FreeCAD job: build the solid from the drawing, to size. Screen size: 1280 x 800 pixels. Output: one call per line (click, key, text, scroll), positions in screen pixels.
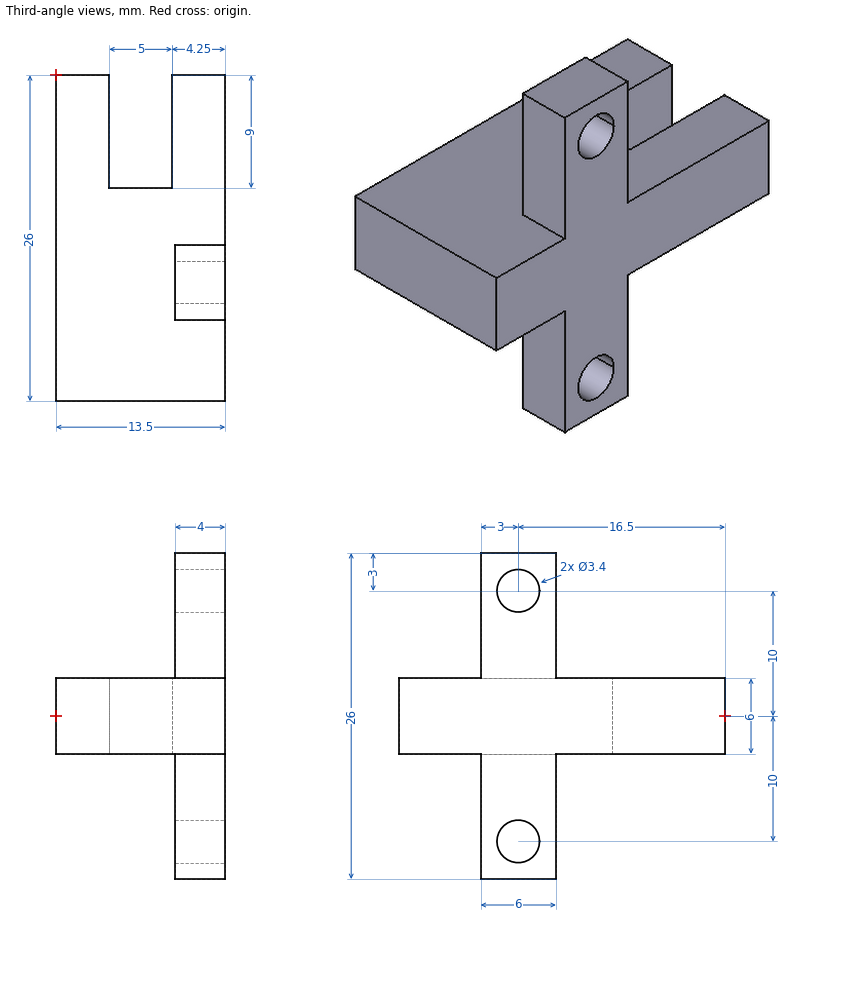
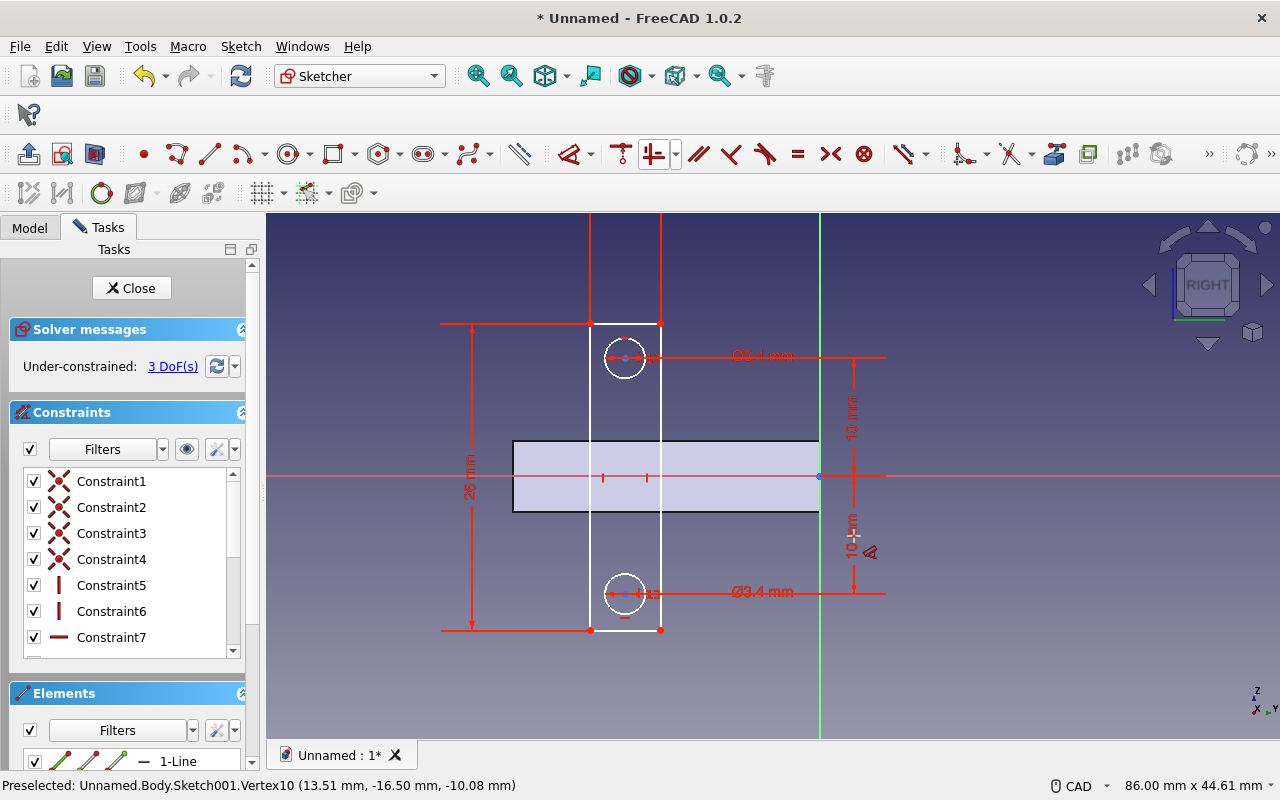
click(590, 324)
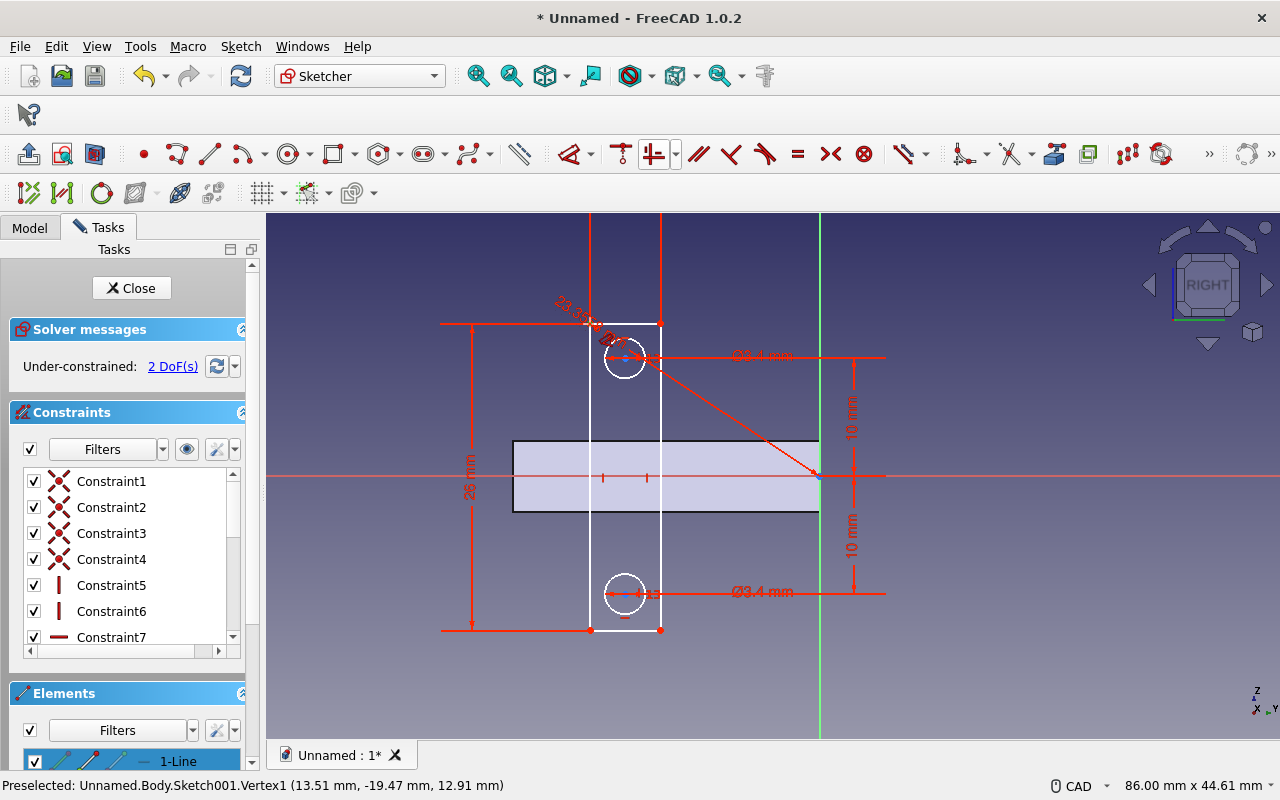
click(625, 358)
click(607, 290)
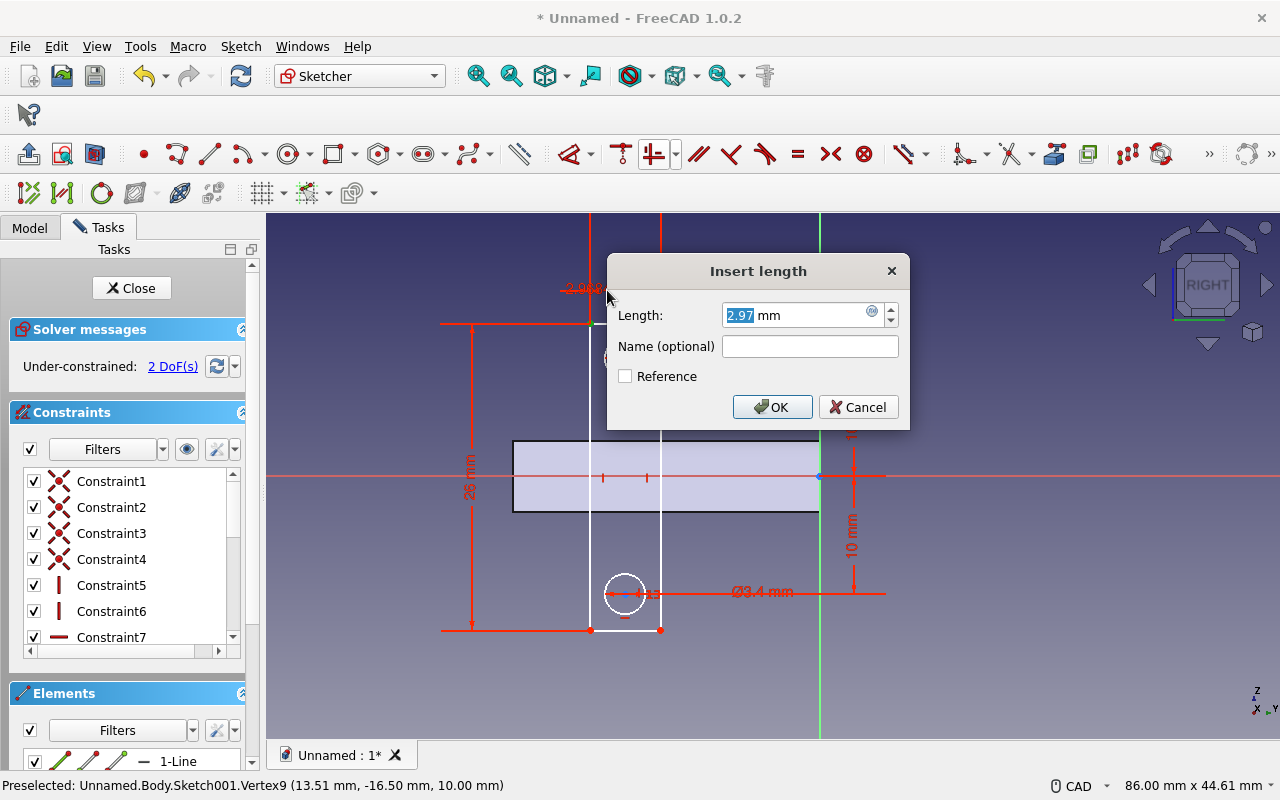
text(3)
key(Return)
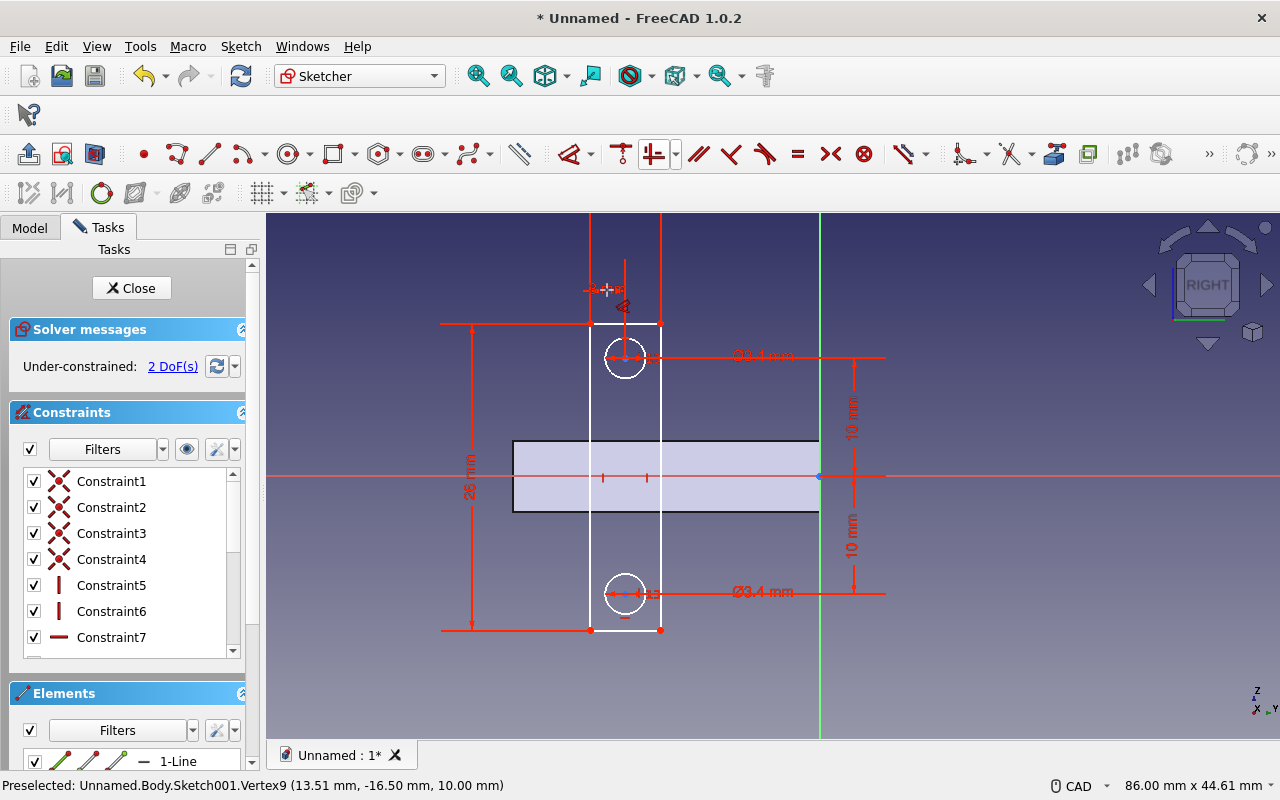
click(590, 324)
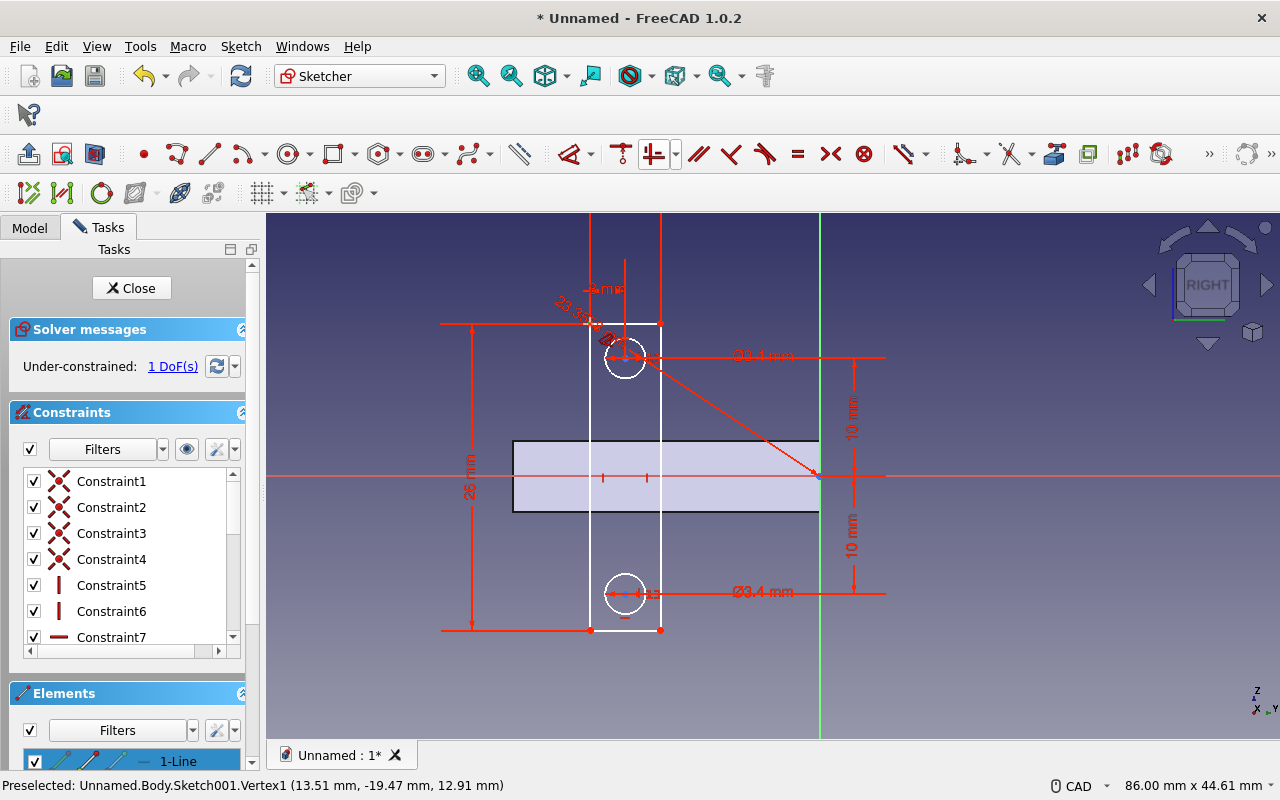
click(625, 358)
click(556, 341)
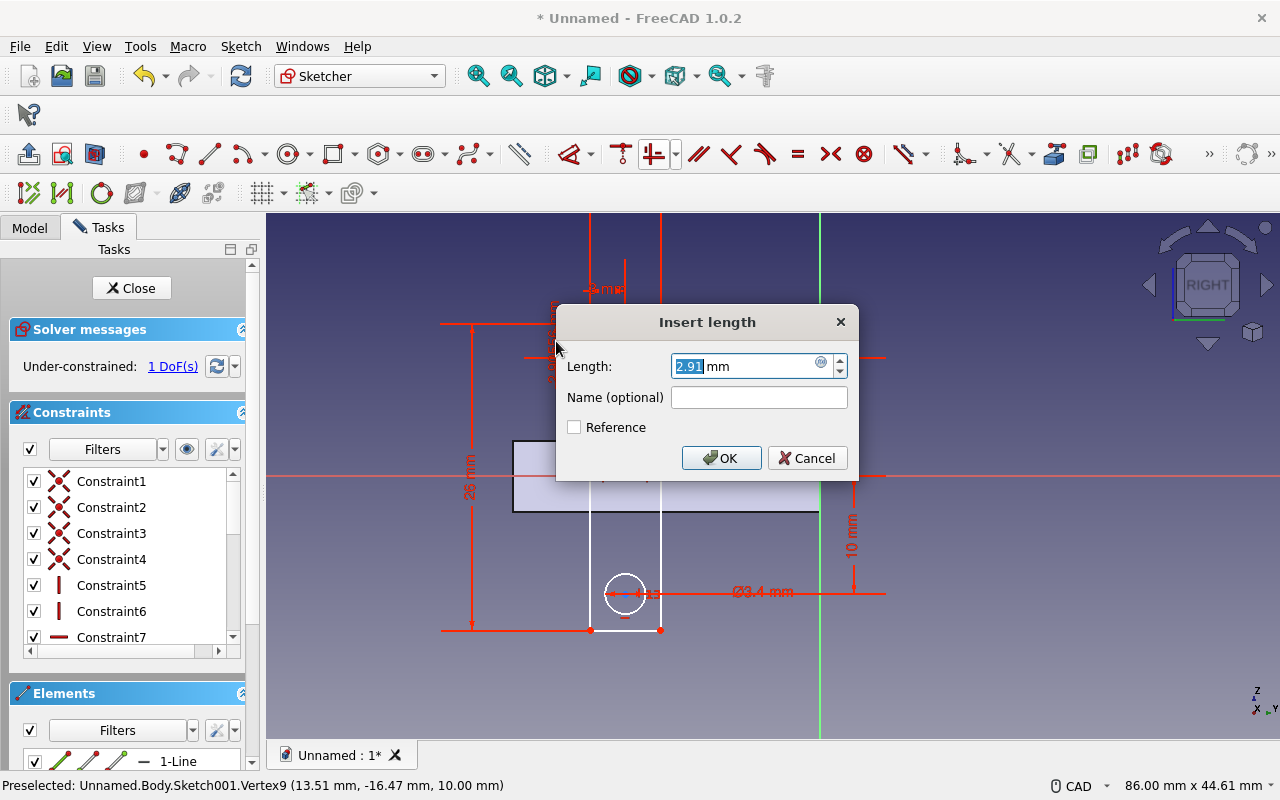
text(3)
key(Return)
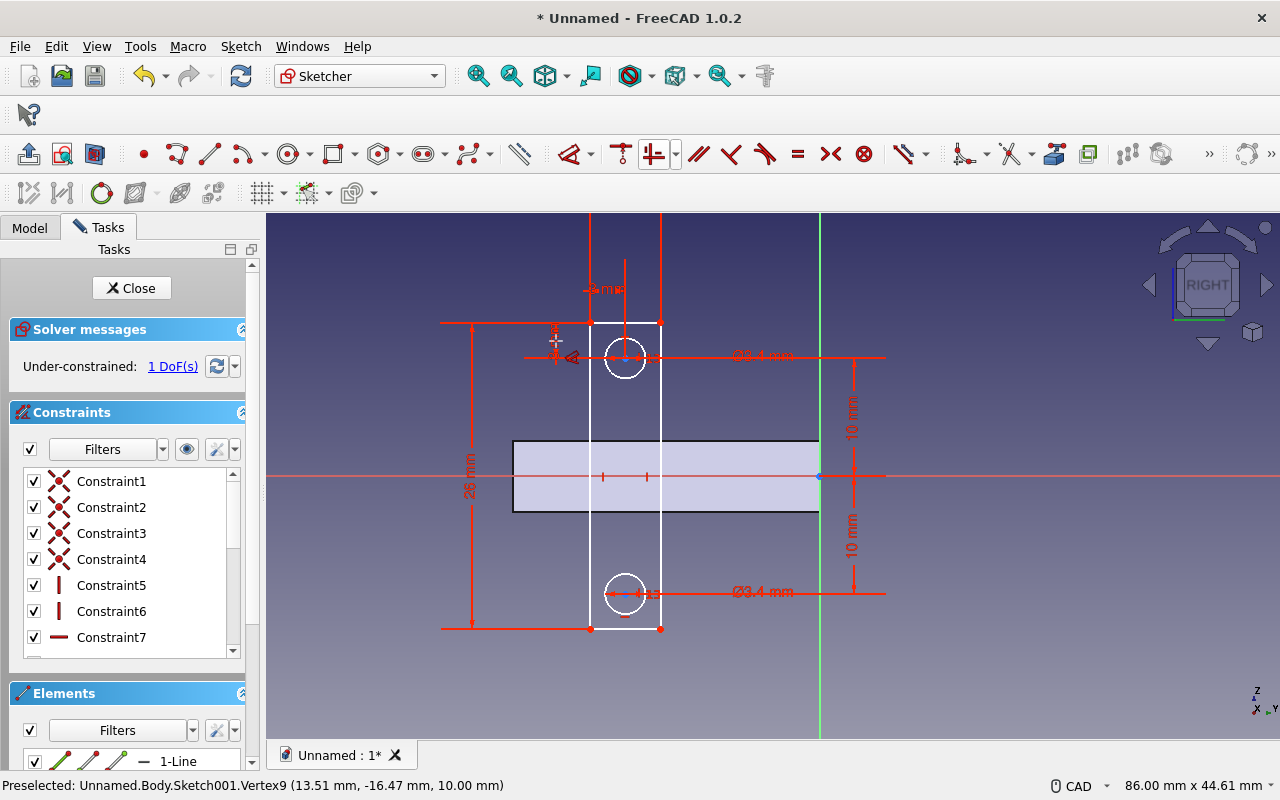
click(625, 358)
click(722, 324)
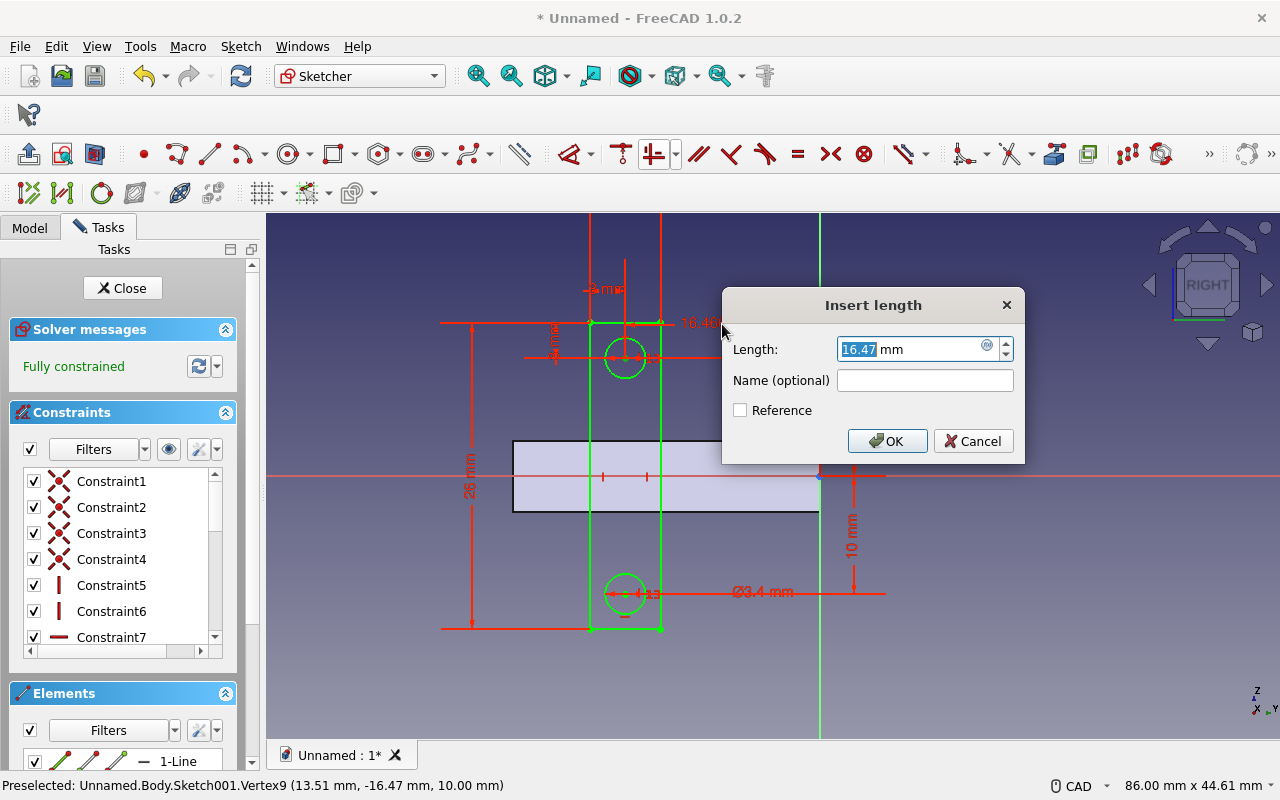
text(16.5)
key(Return)
key(Escape)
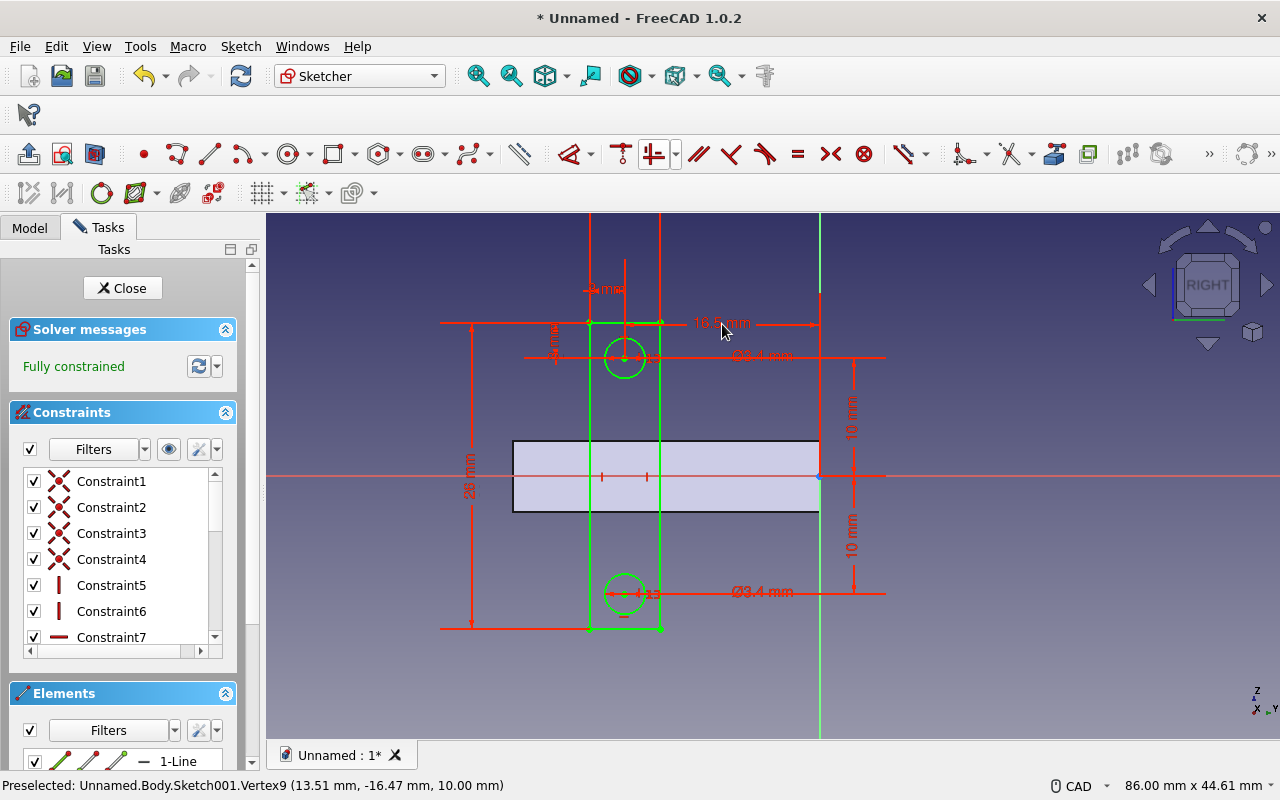
click(123, 288)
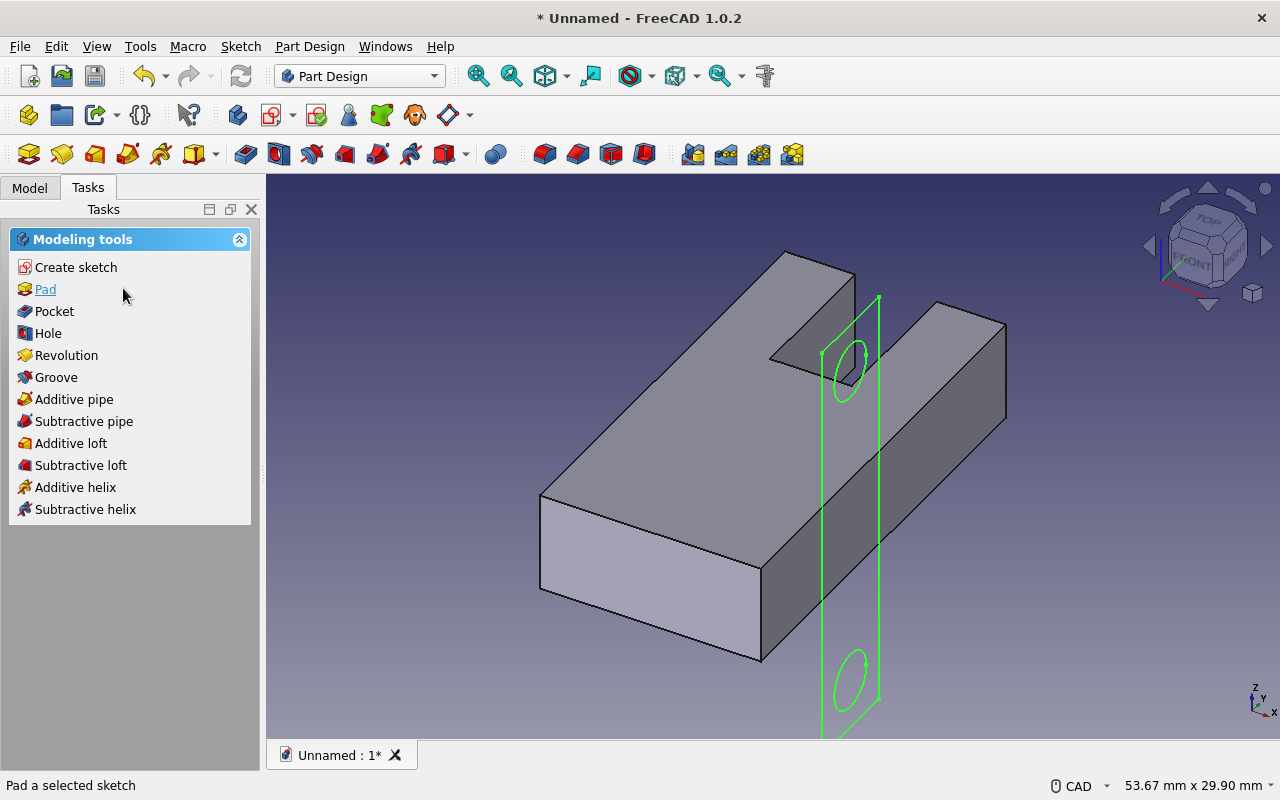
click(29, 154)